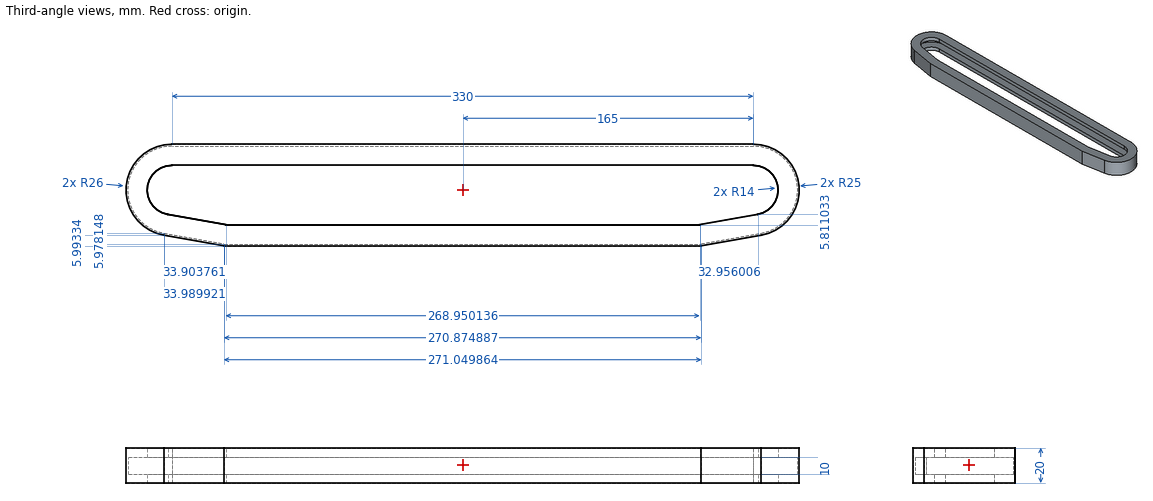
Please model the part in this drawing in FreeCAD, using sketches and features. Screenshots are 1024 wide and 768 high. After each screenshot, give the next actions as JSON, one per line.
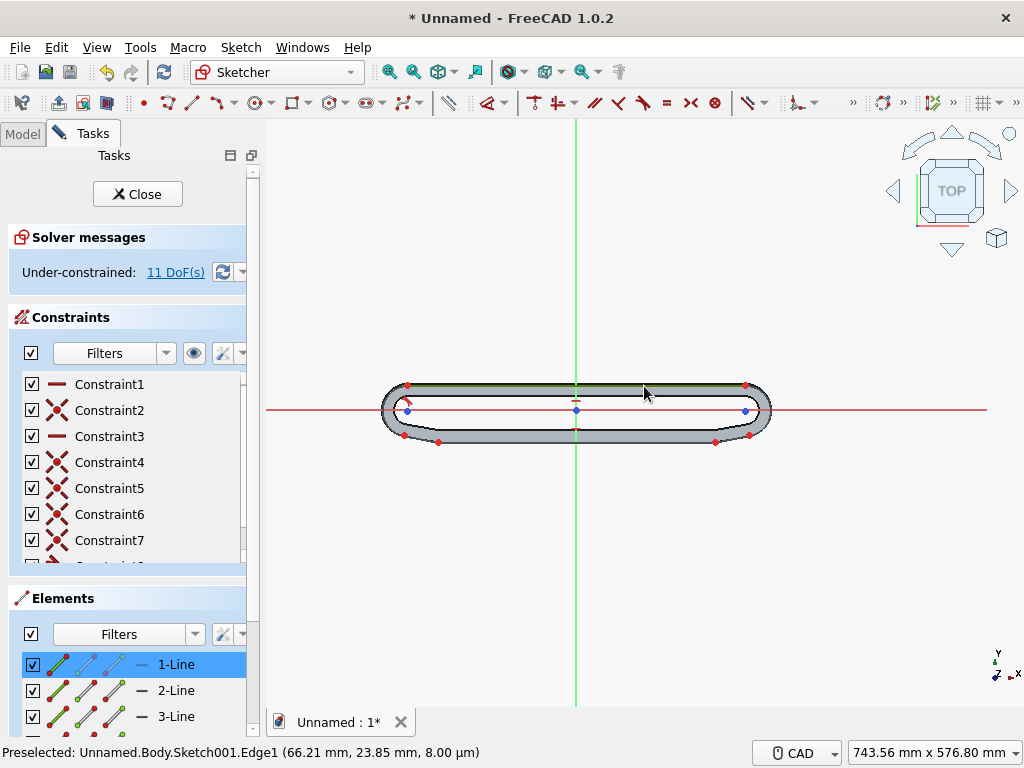
{"action": "left_click", "coordinate": [767, 424]}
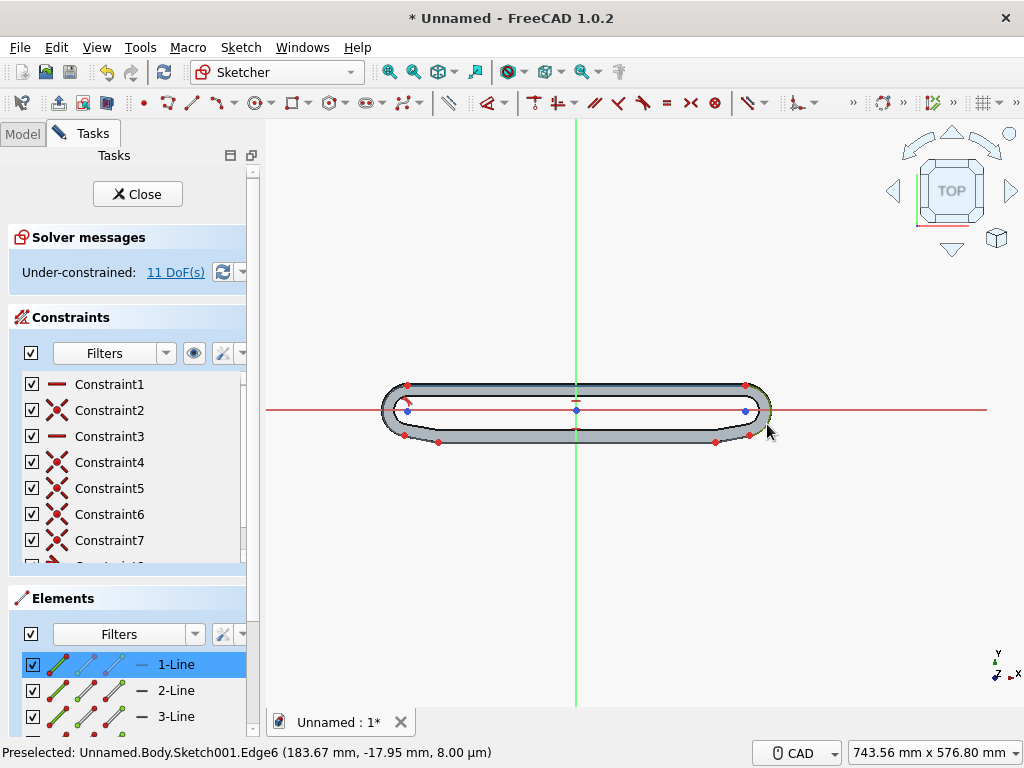
{"action": "left_click", "coordinate": [644, 104]}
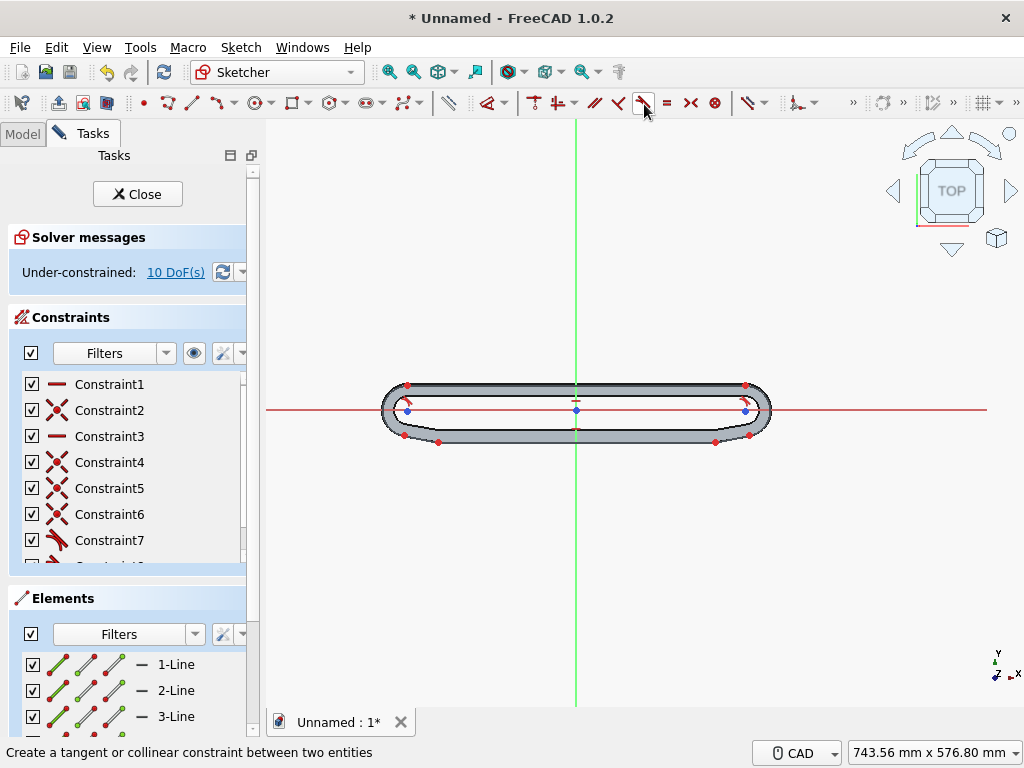
{"action": "scroll", "coordinate": [414, 438], "scroll_direction": "up", "scroll_amount": 2}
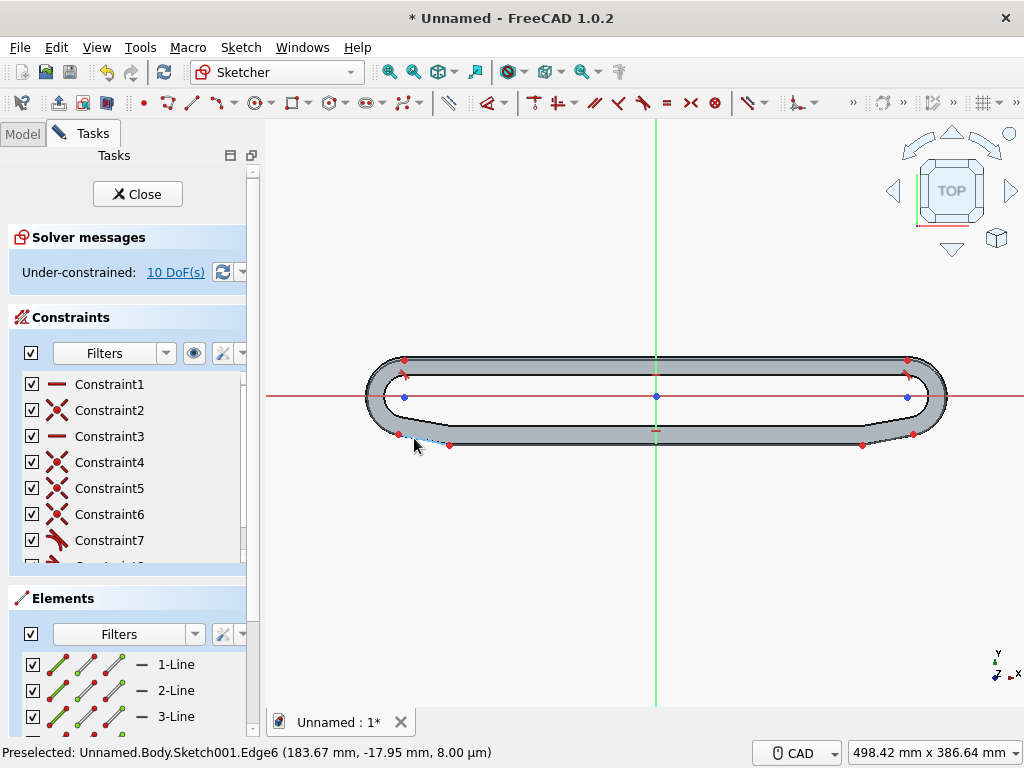
{"action": "left_click", "coordinate": [414, 438]}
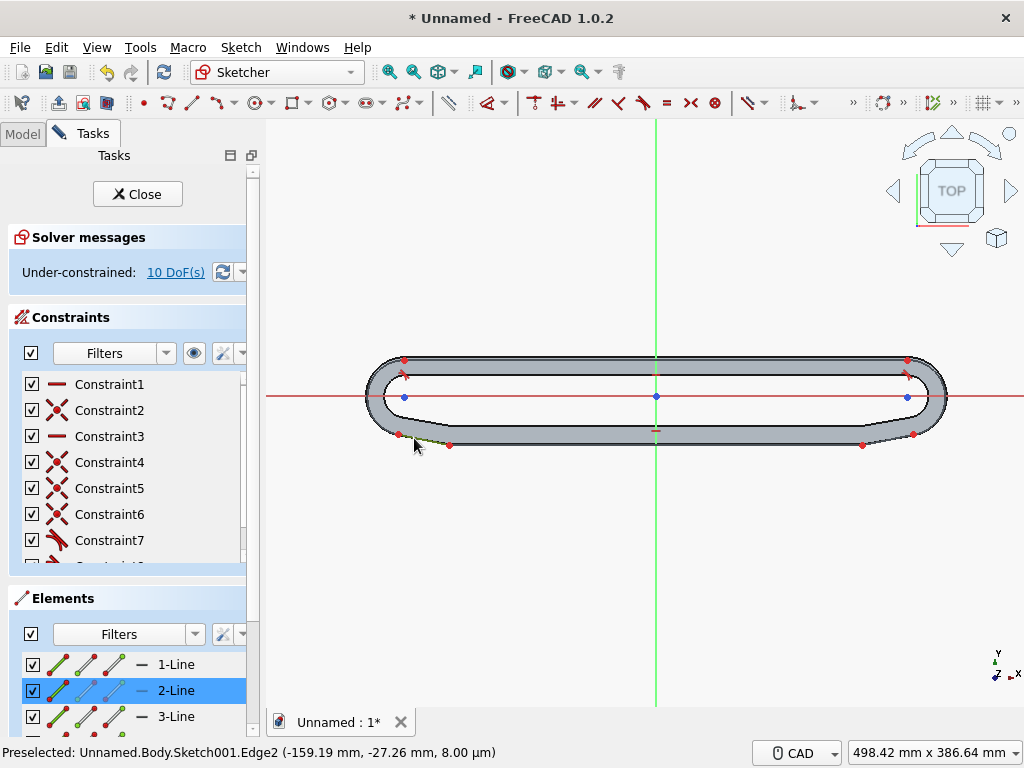
{"action": "left_click", "coordinate": [376, 374]}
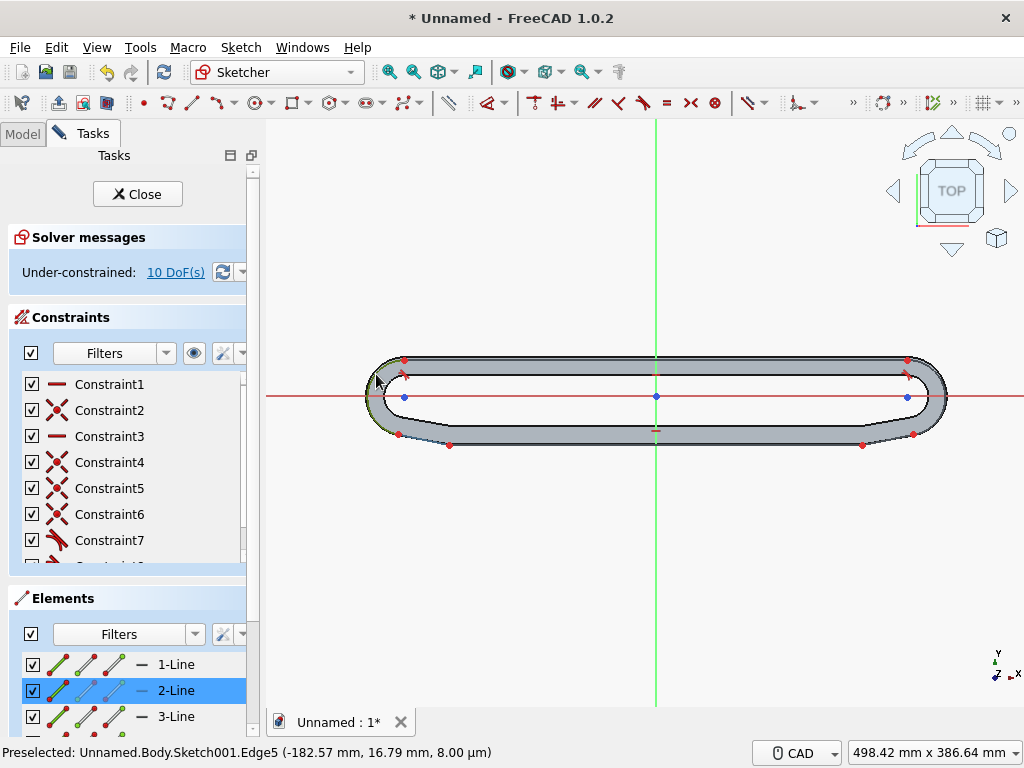
{"action": "left_click", "coordinate": [644, 104]}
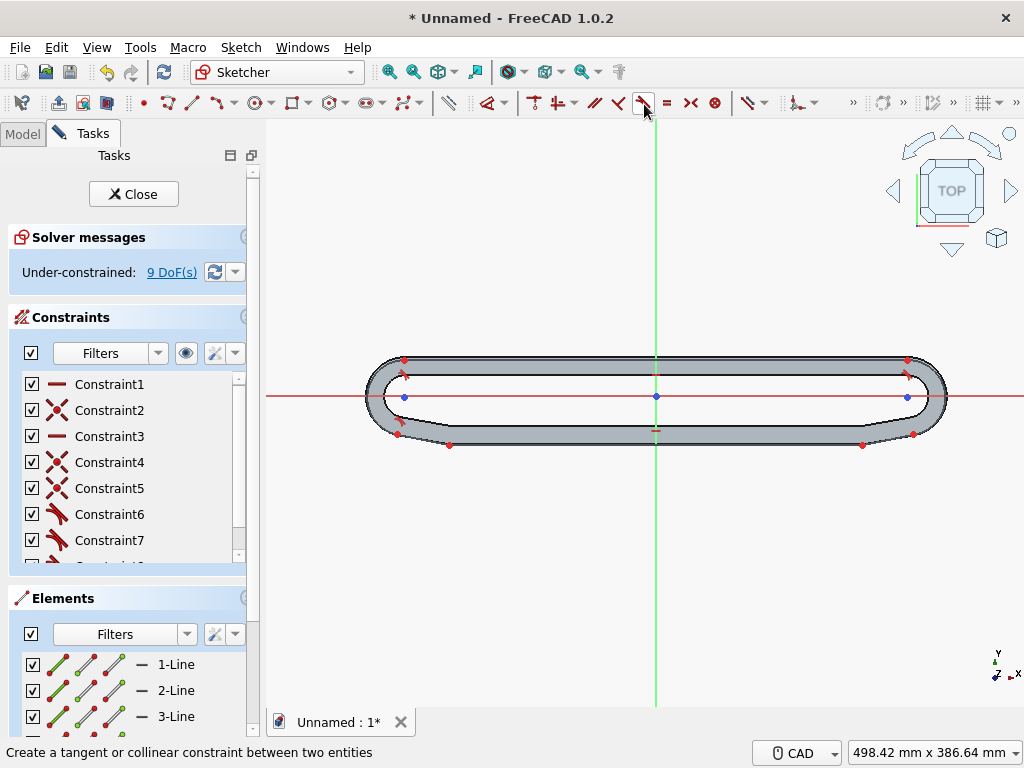
{"action": "scroll", "coordinate": [414, 438], "scroll_direction": "down", "scroll_amount": 2}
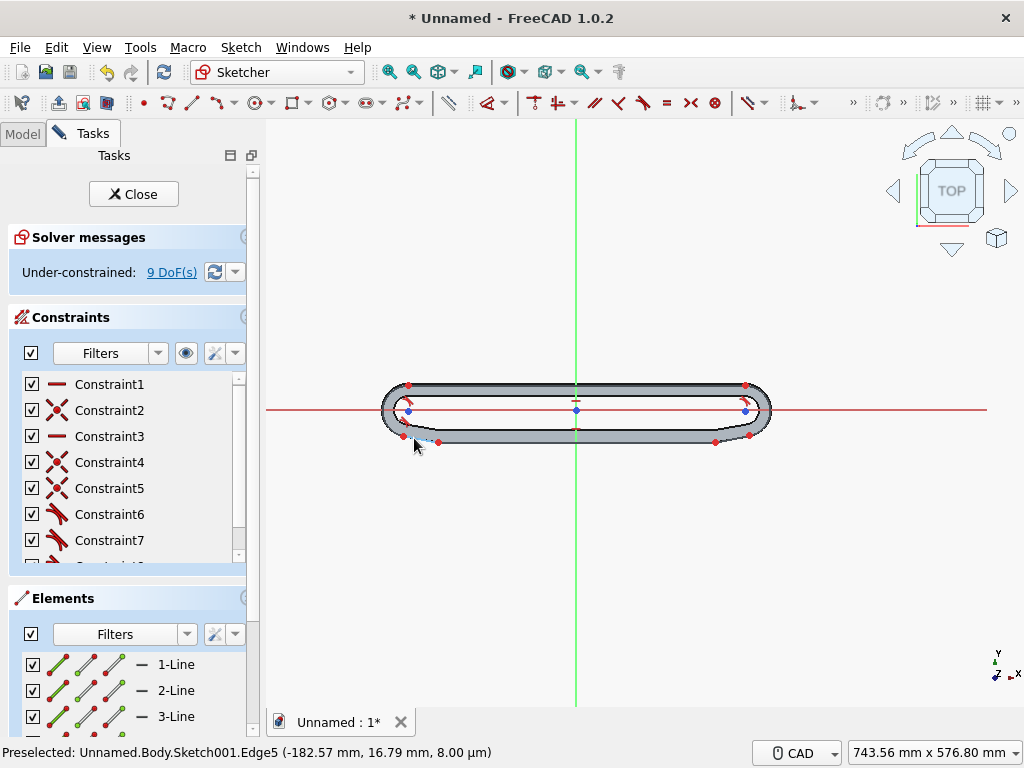
{"action": "scroll", "coordinate": [725, 441], "scroll_direction": "up", "scroll_amount": 2}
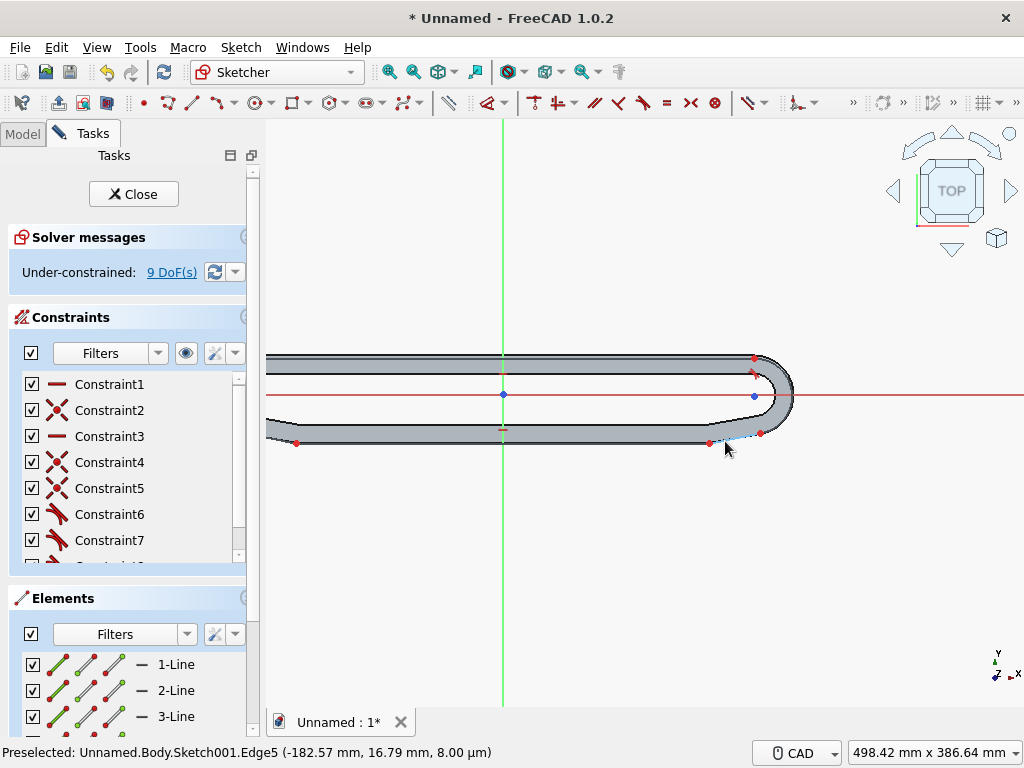
{"action": "left_click", "coordinate": [725, 441]}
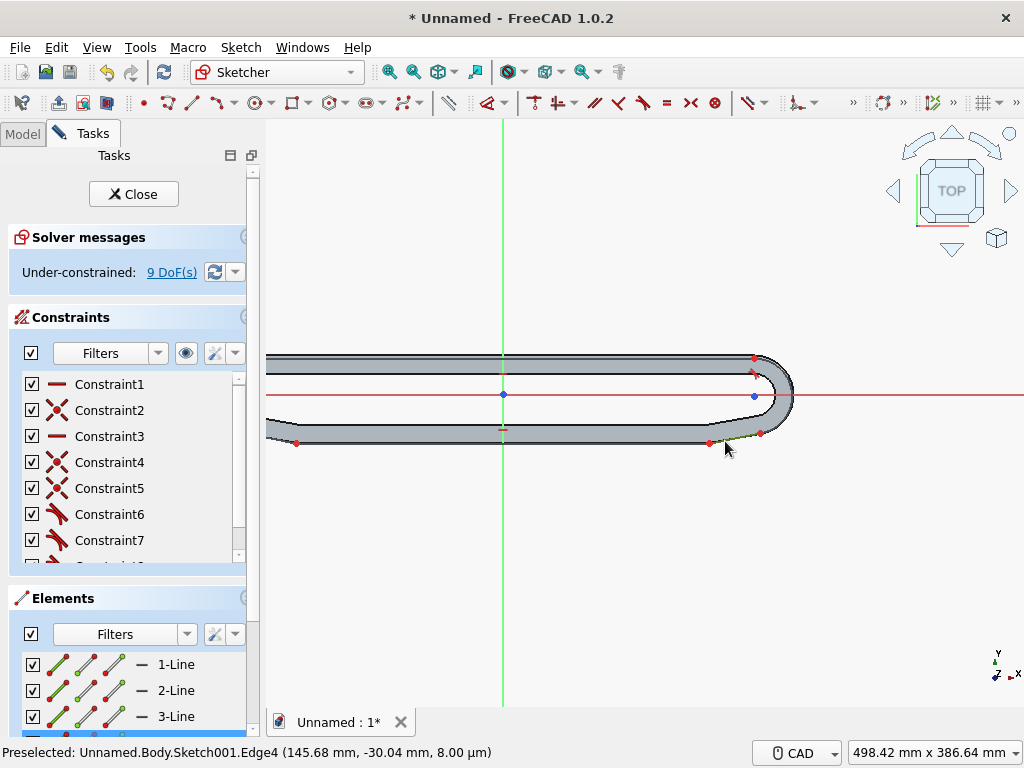
{"action": "left_click", "coordinate": [787, 415]}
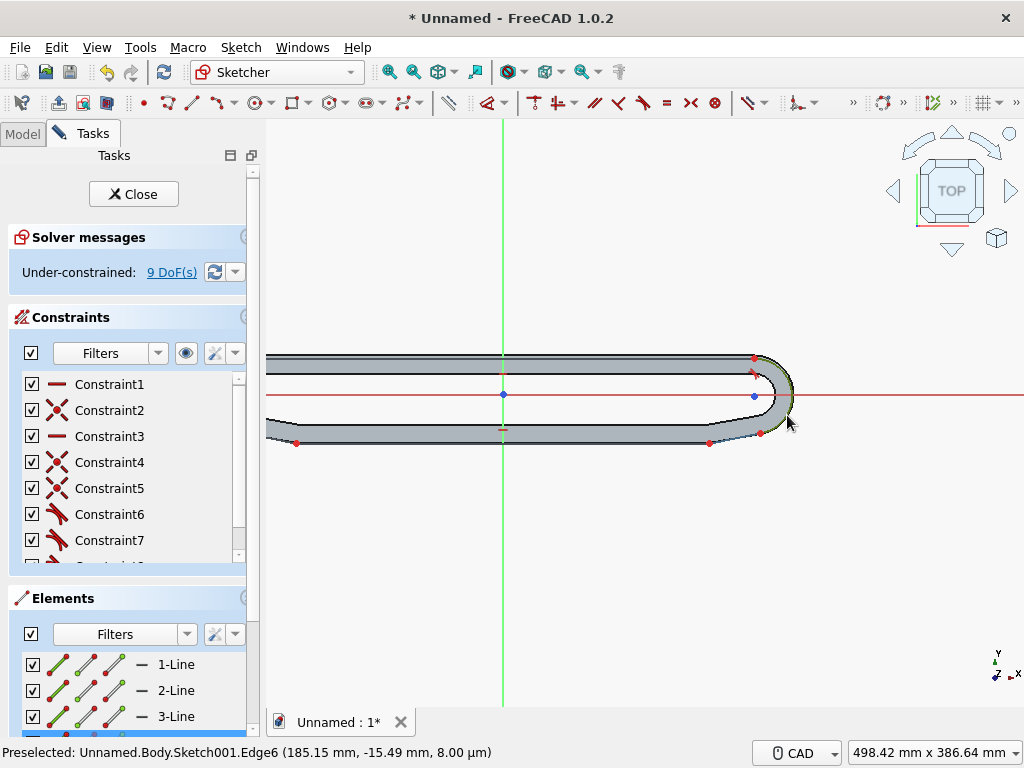
{"action": "left_click", "coordinate": [644, 104]}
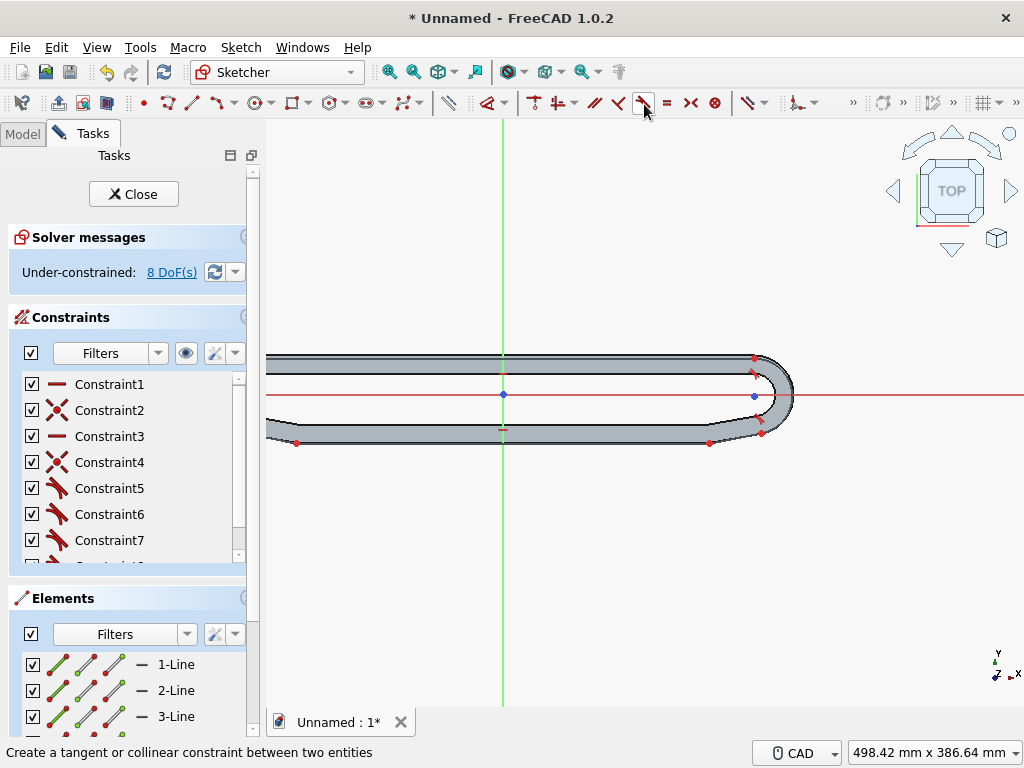
{"action": "scroll", "coordinate": [726, 441], "scroll_direction": "down", "scroll_amount": 2}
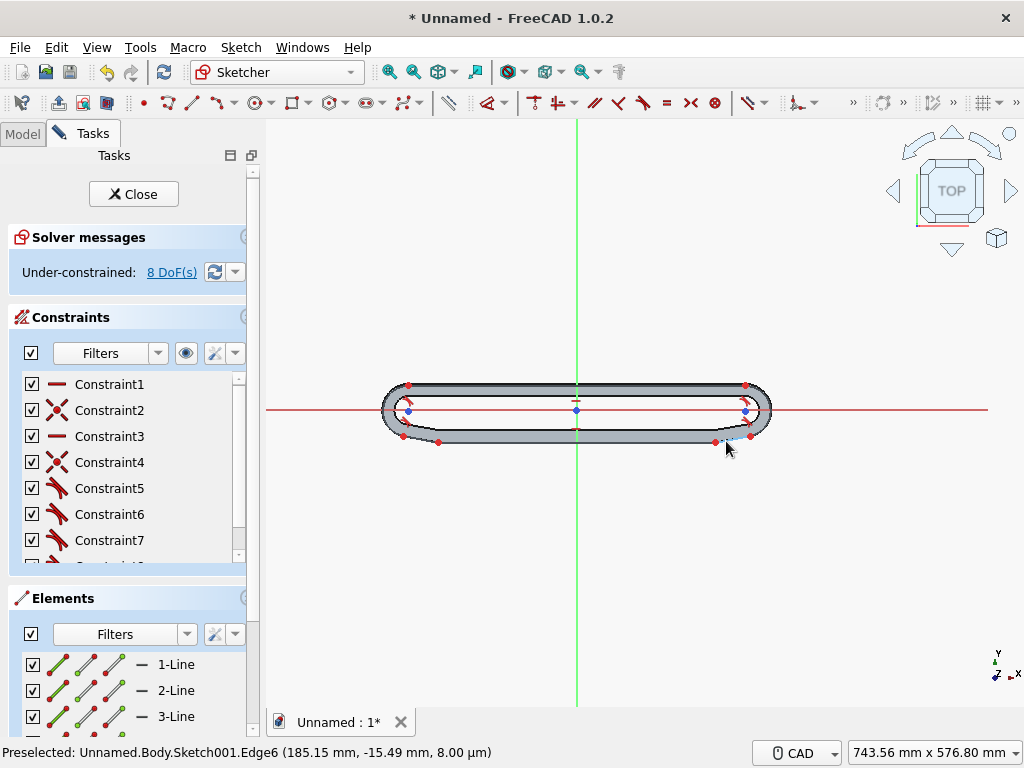
{"action": "left_click", "coordinate": [389, 395]}